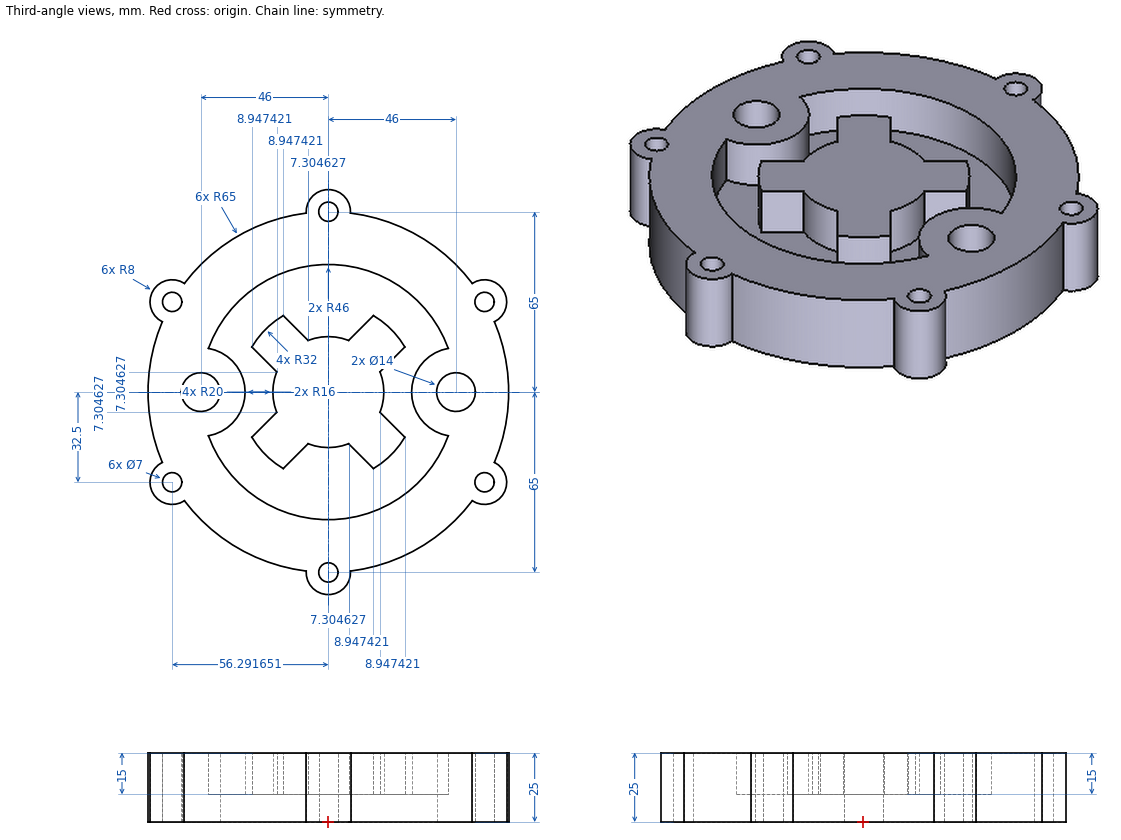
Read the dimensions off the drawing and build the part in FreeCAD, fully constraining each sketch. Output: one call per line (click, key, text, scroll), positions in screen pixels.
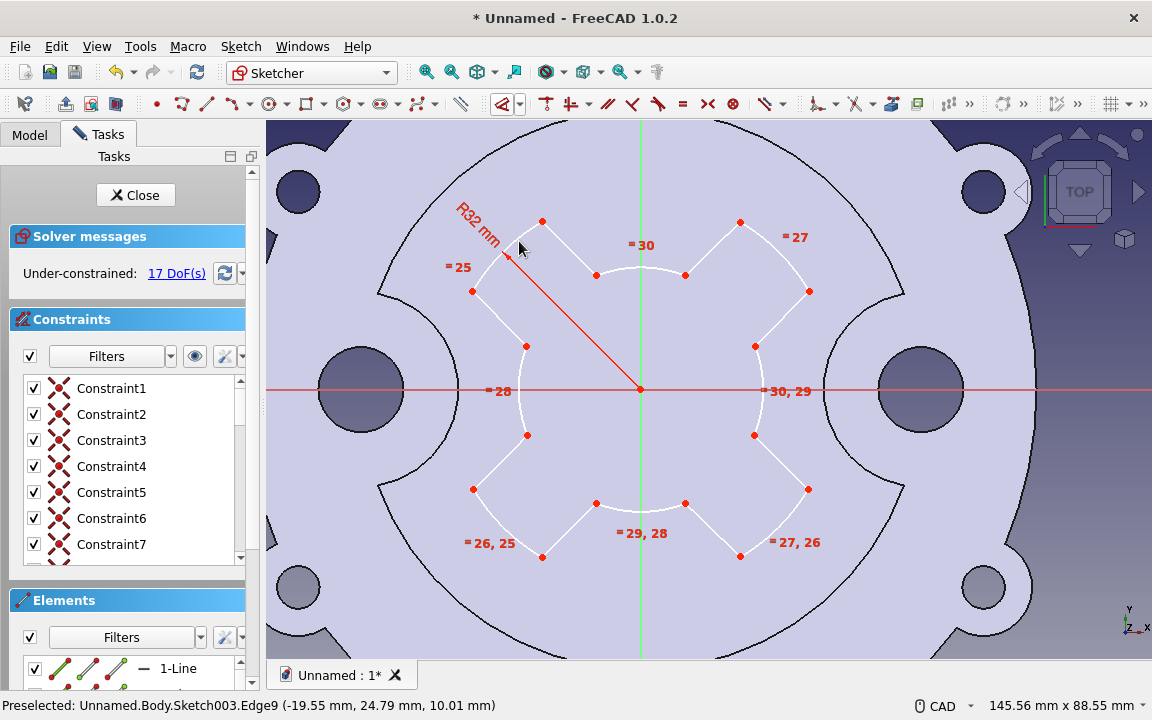
click(520, 373)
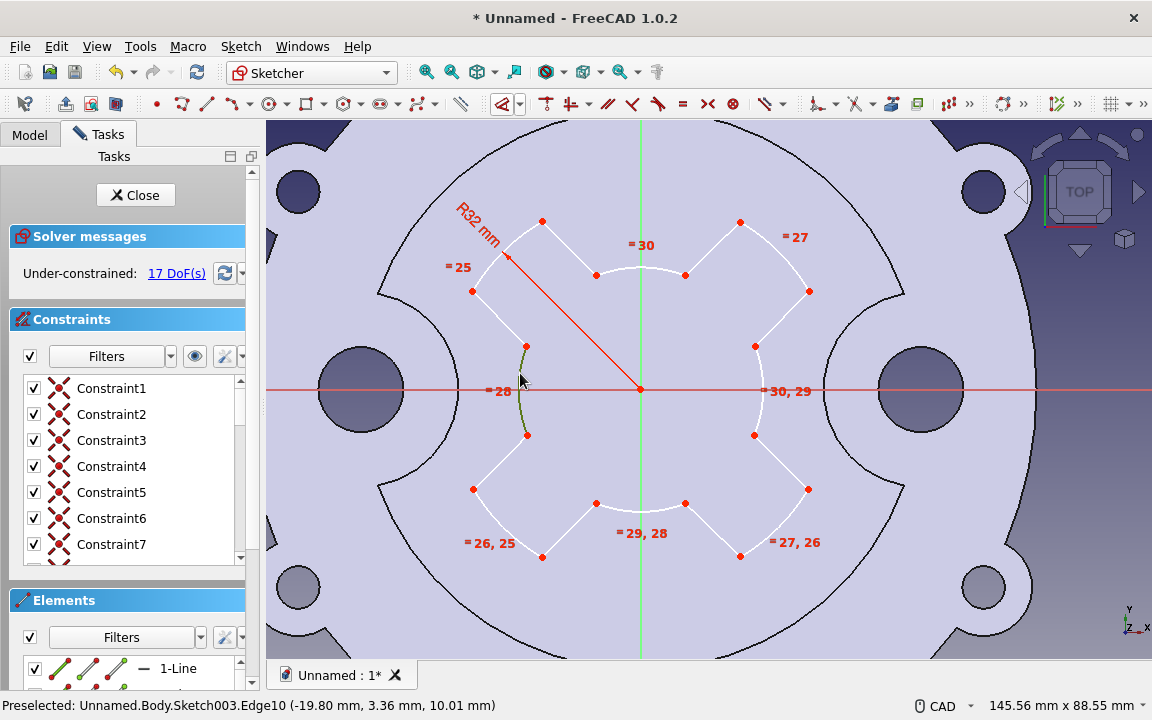
click(520, 104)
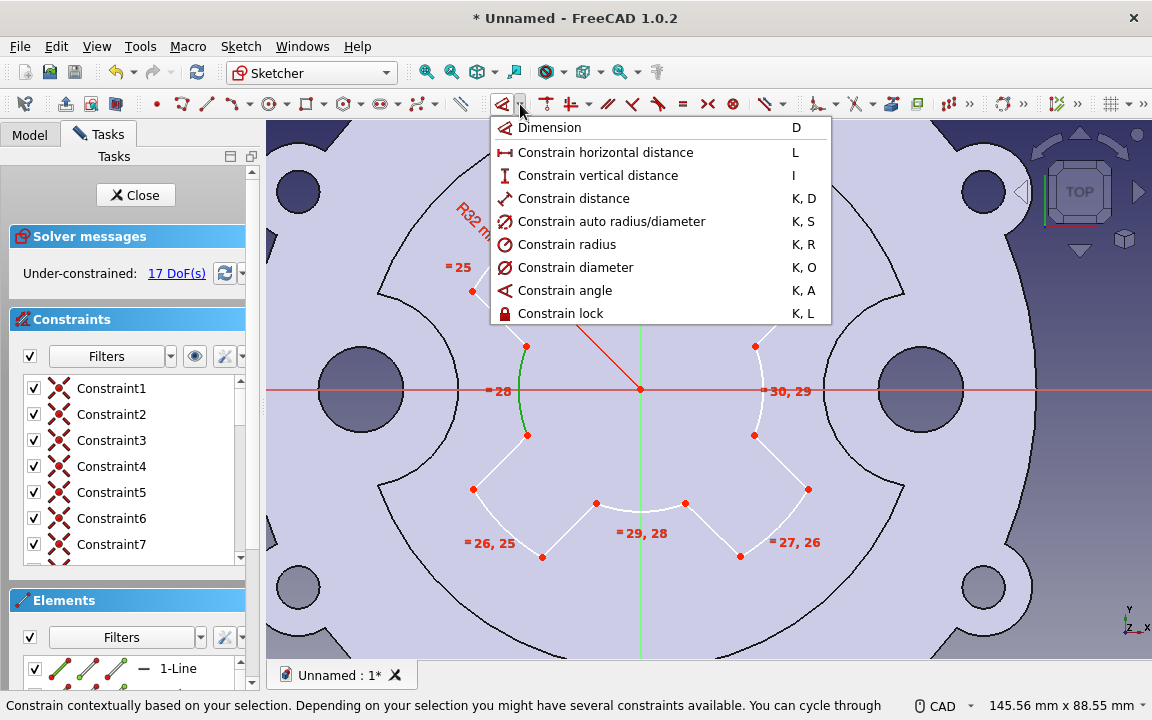
click(661, 244)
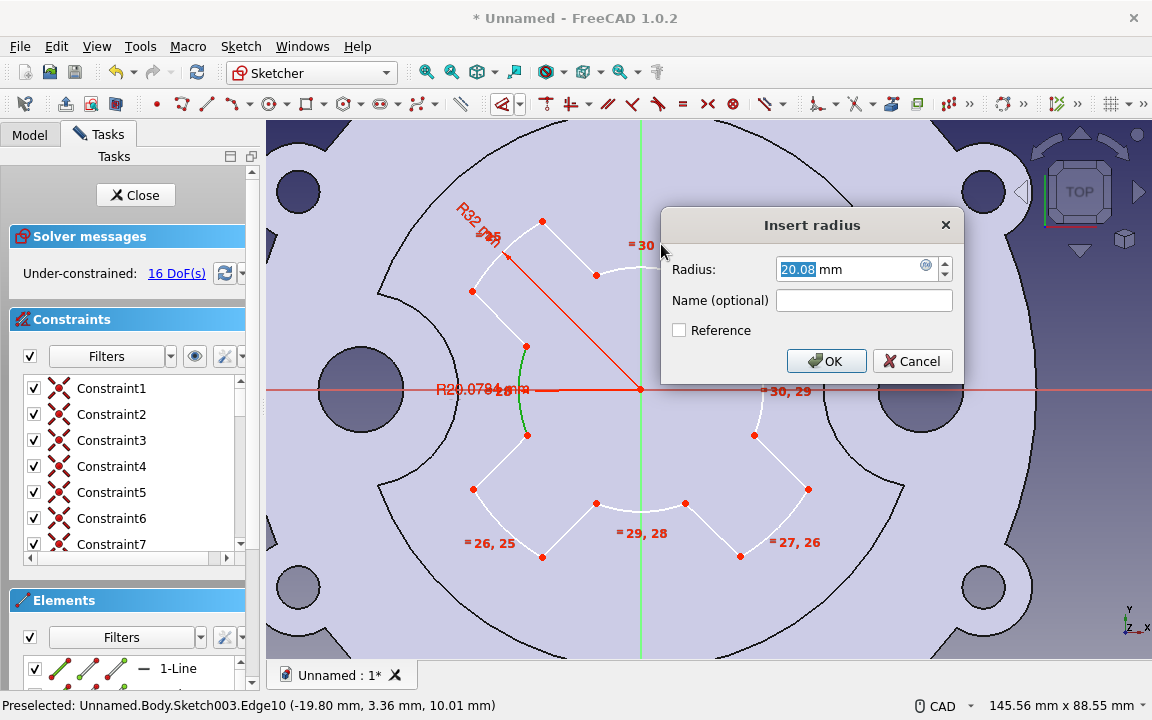
text(20)
key(Return)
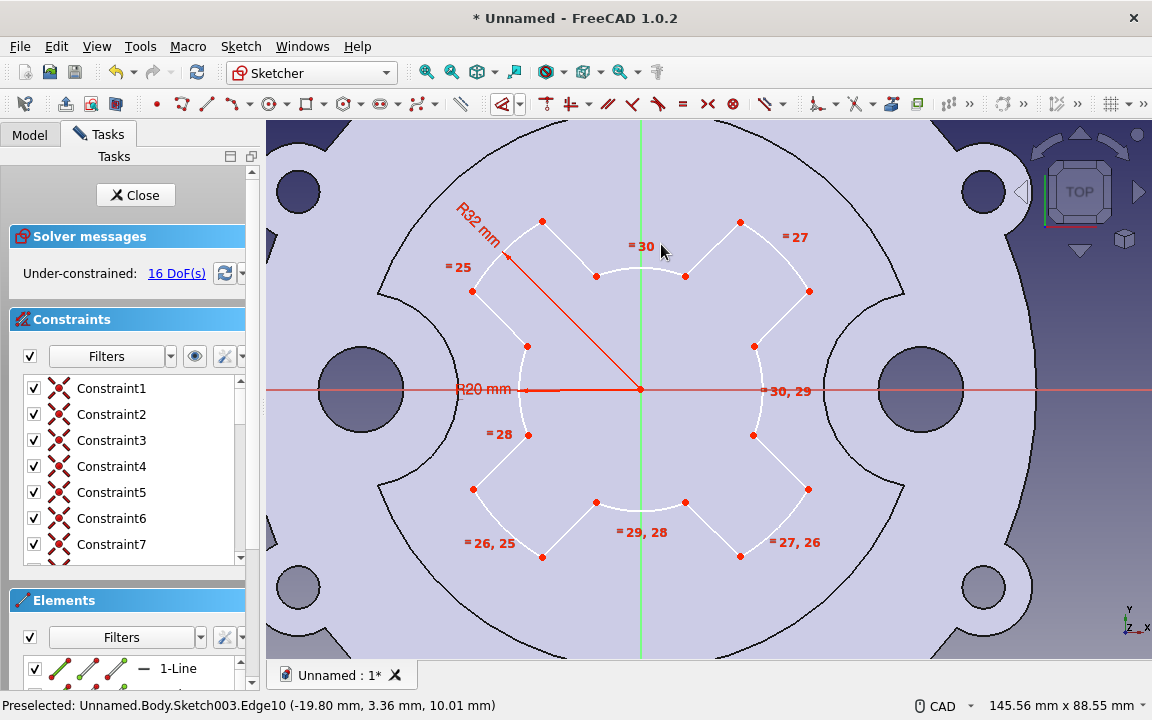
click(596, 276)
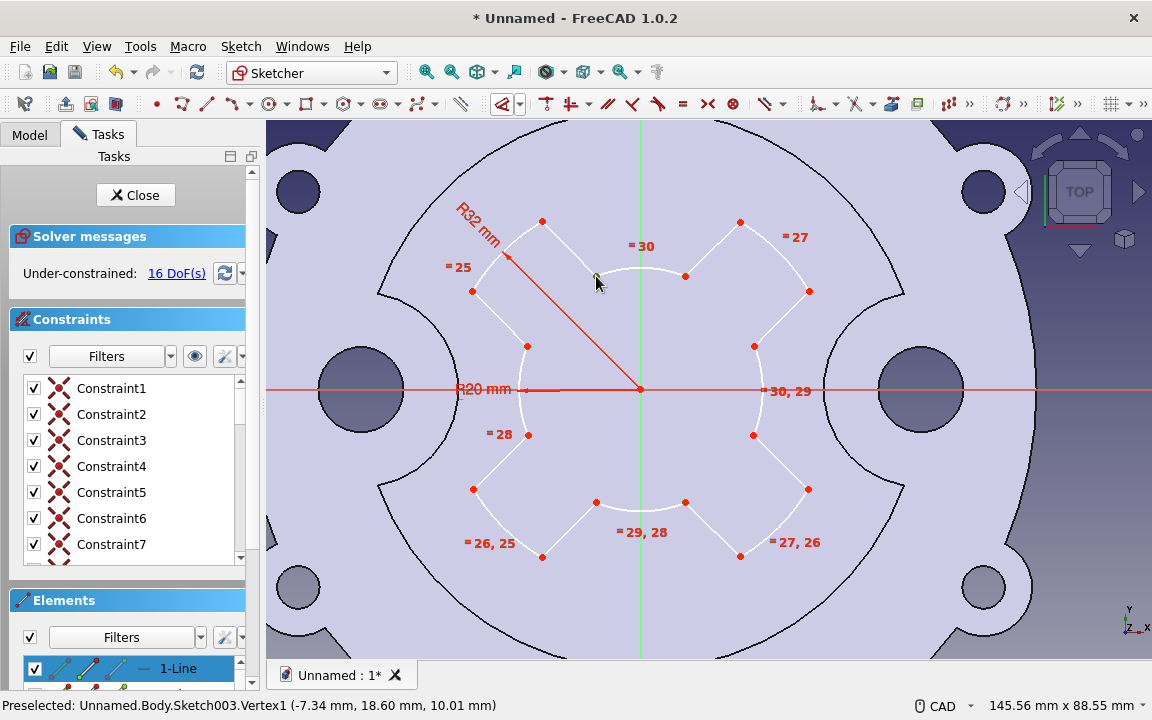
click(520, 104)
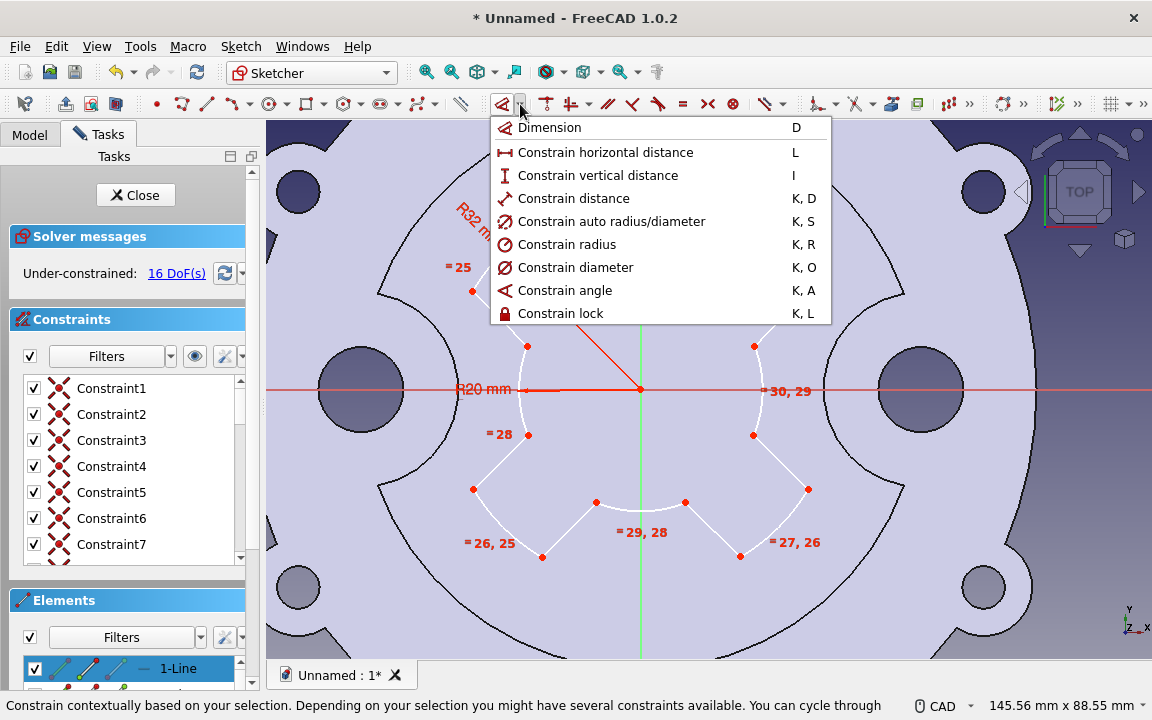
click(661, 152)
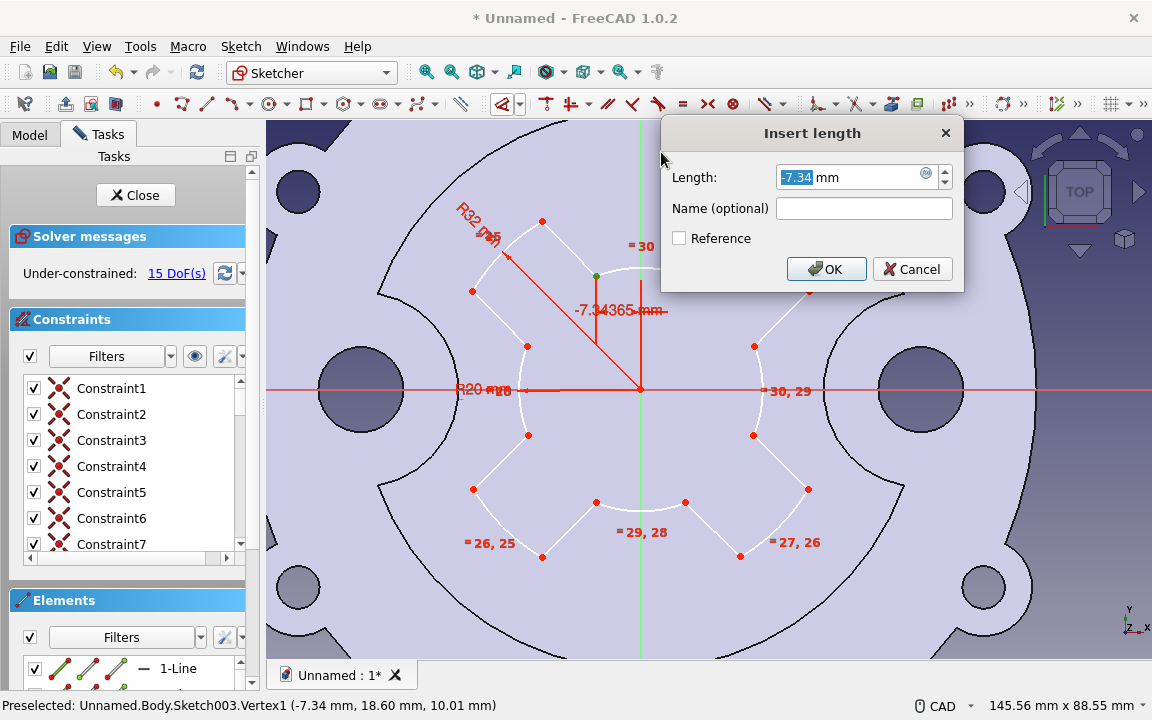
text(-7.304627)
key(Return)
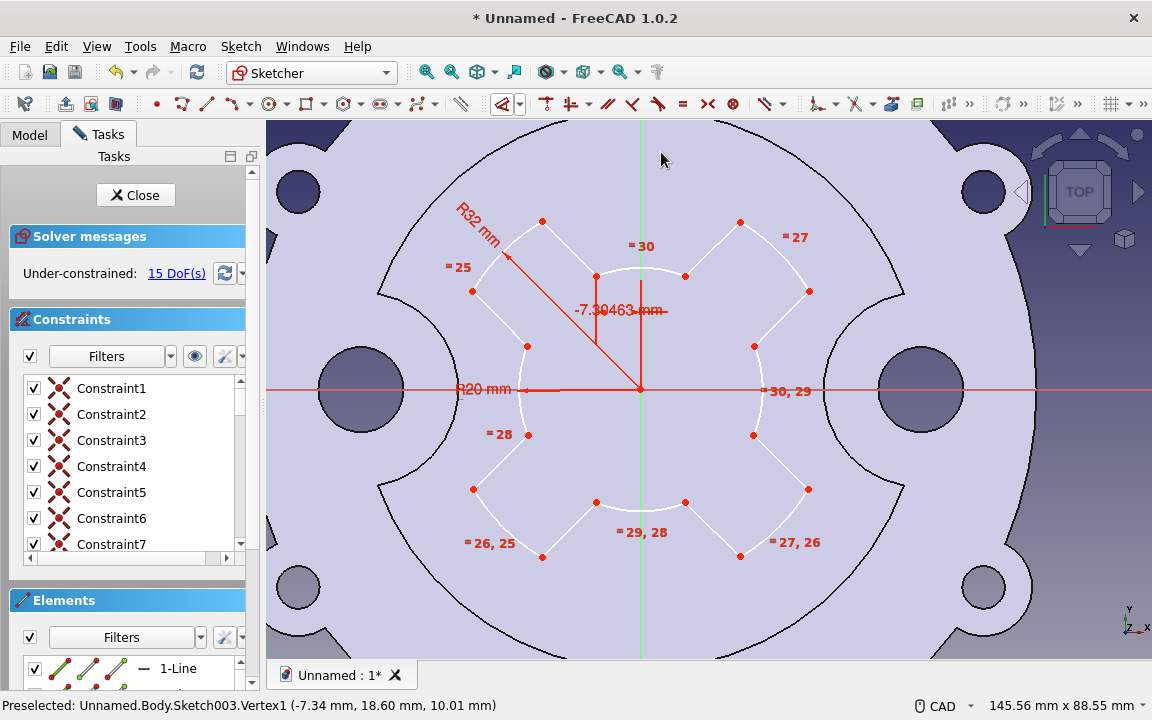
click(527, 346)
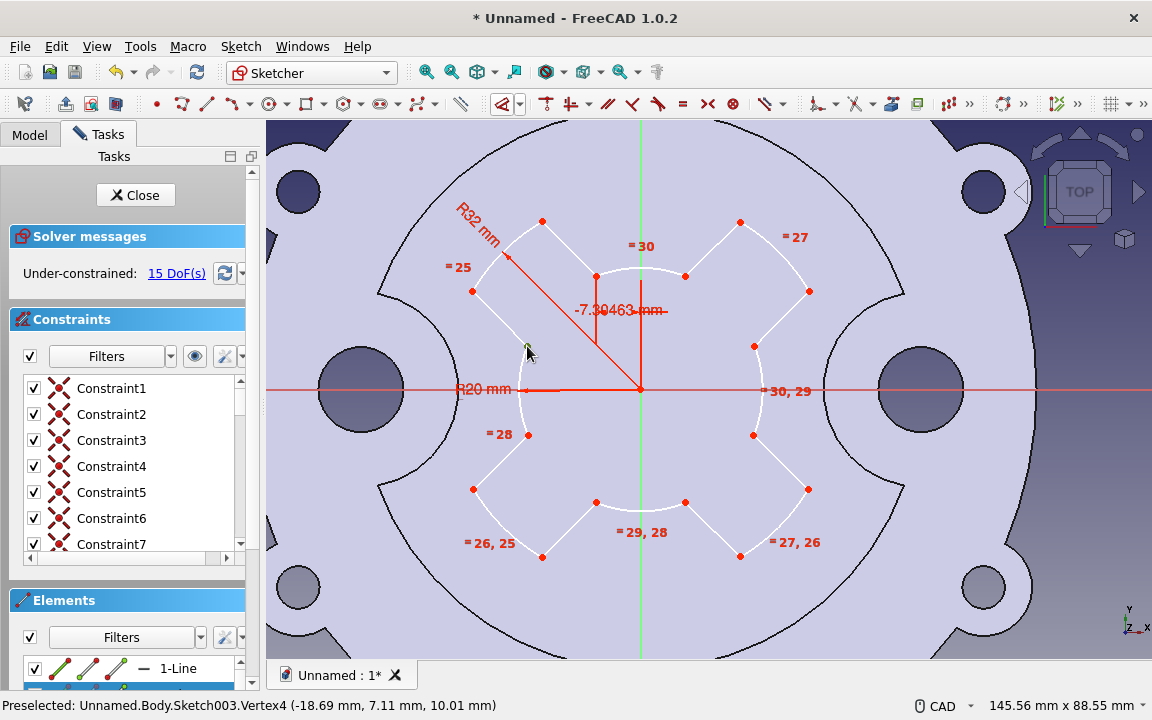
click(520, 104)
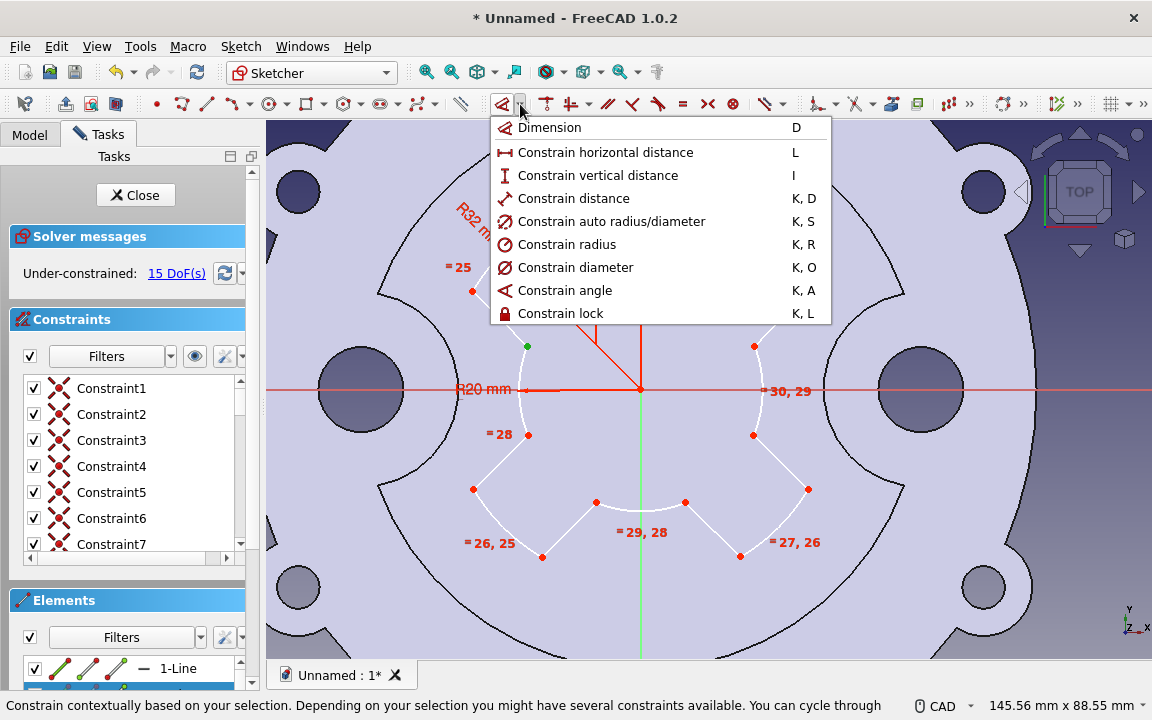
click(661, 176)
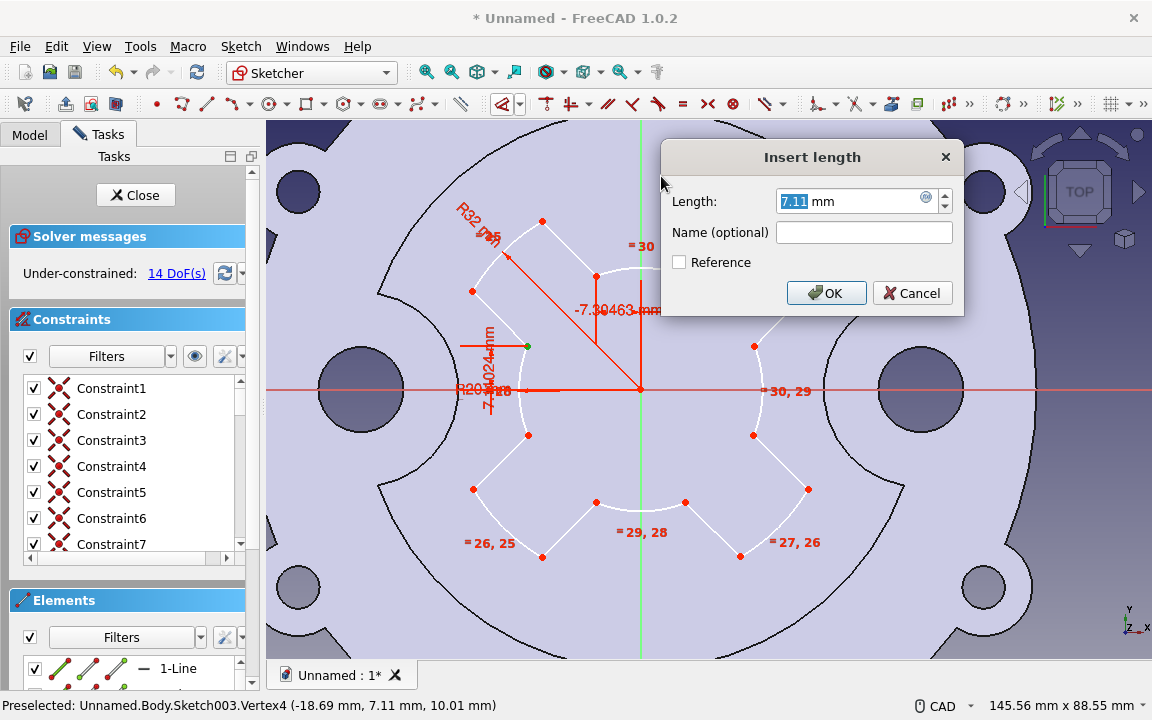
text(7.304627)
key(Return)